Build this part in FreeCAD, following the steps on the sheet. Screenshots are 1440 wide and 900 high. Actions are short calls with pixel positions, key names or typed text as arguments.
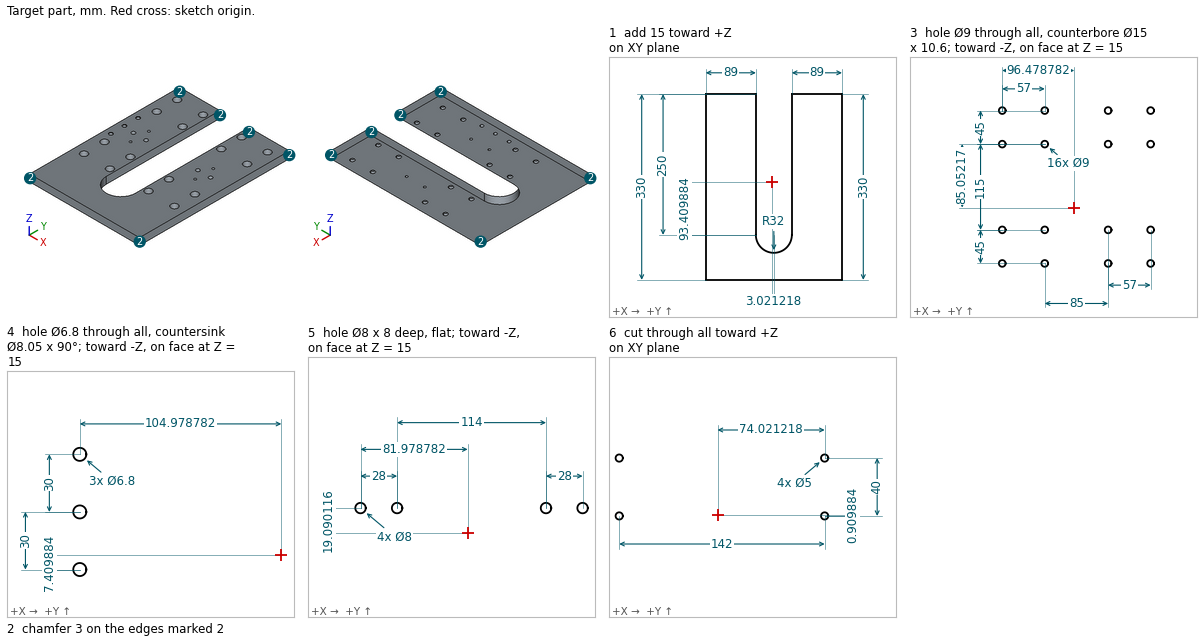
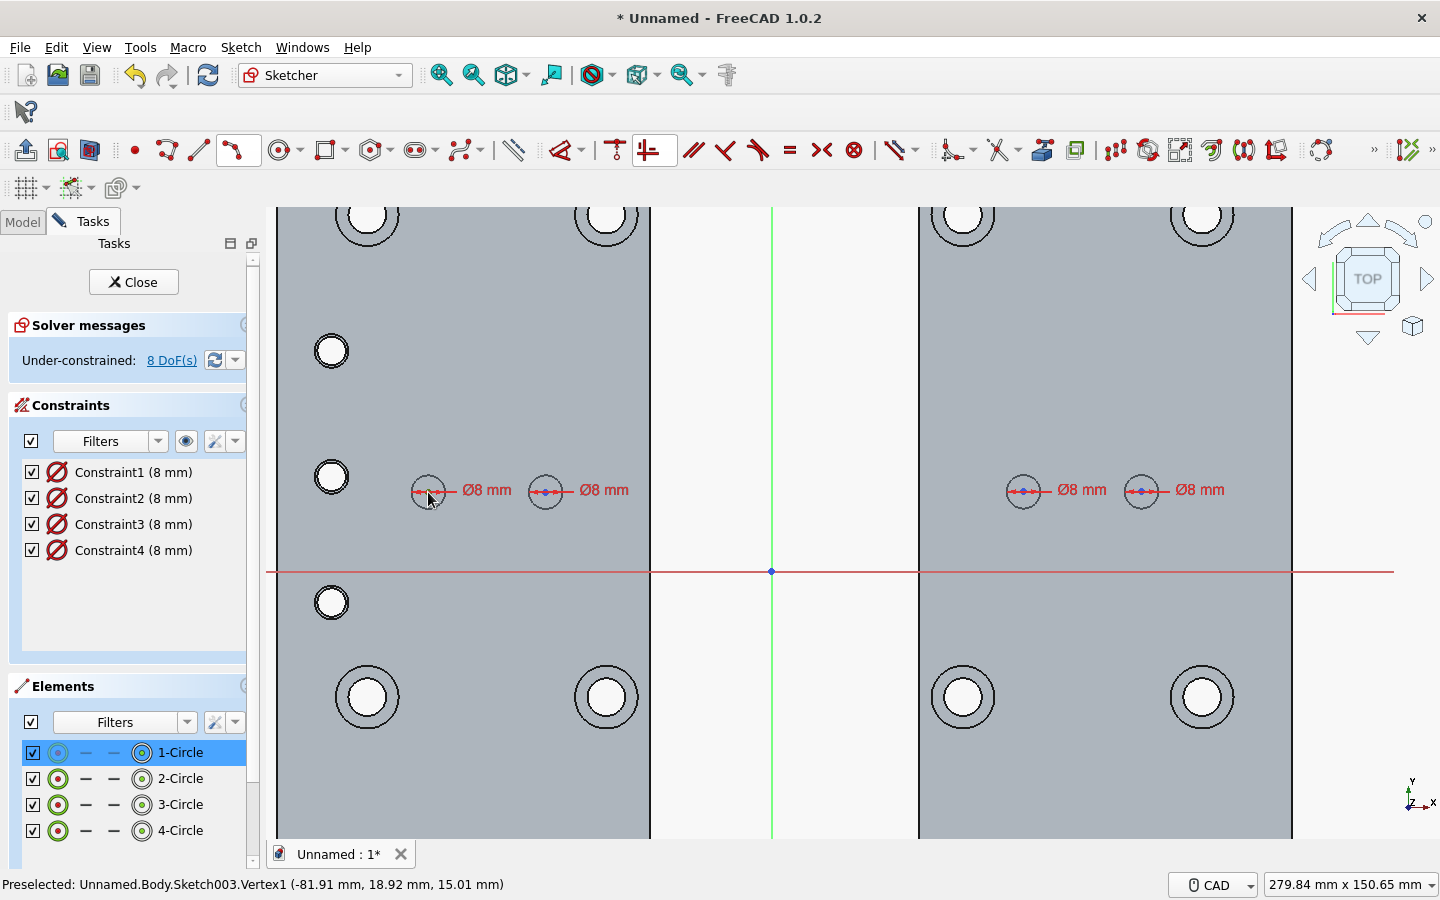
click(546, 492)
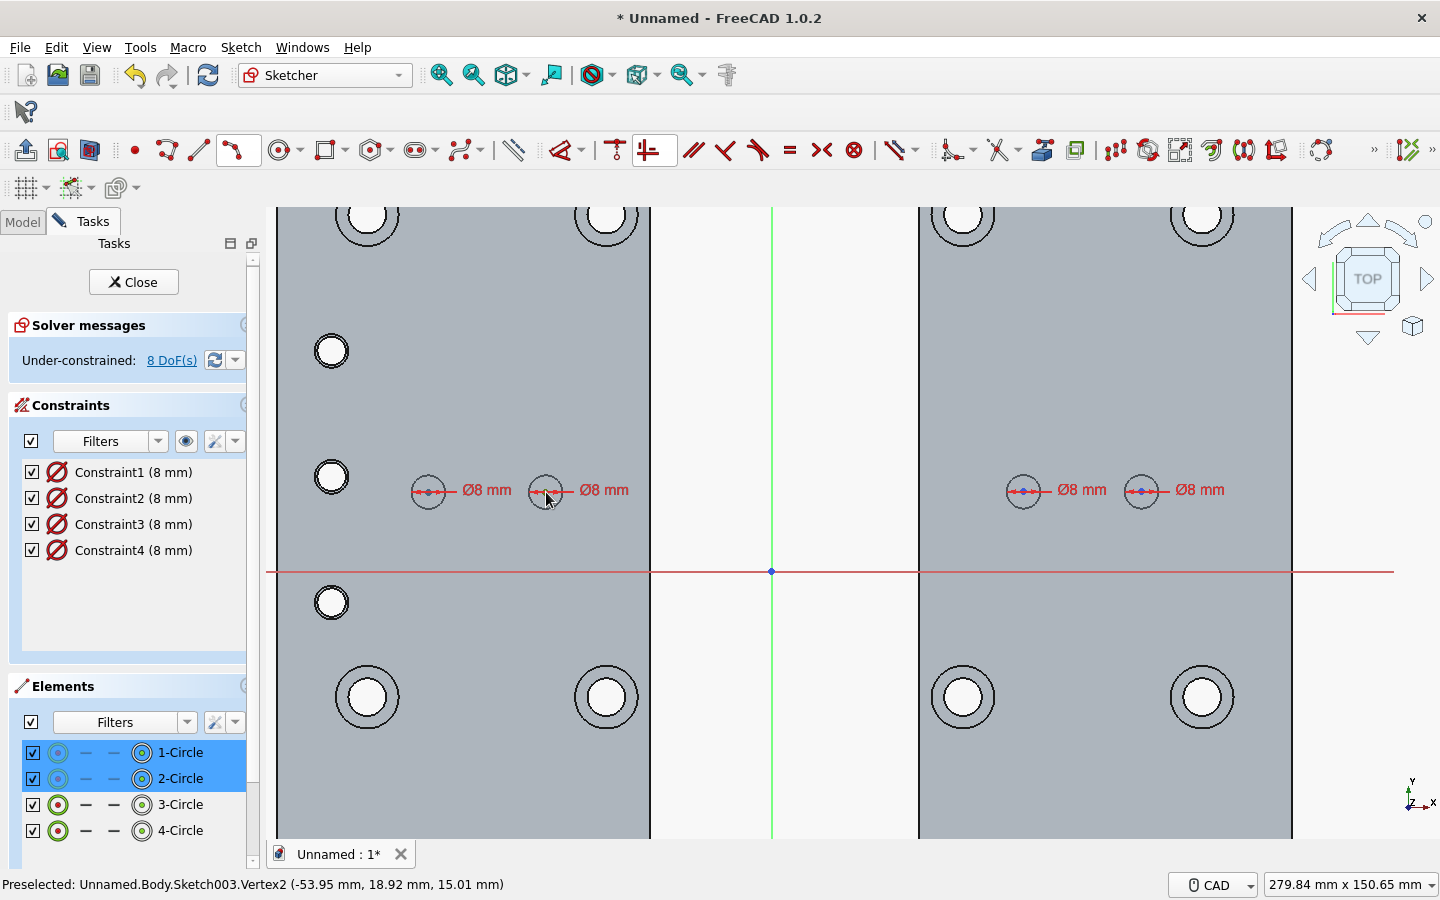
click(672, 150)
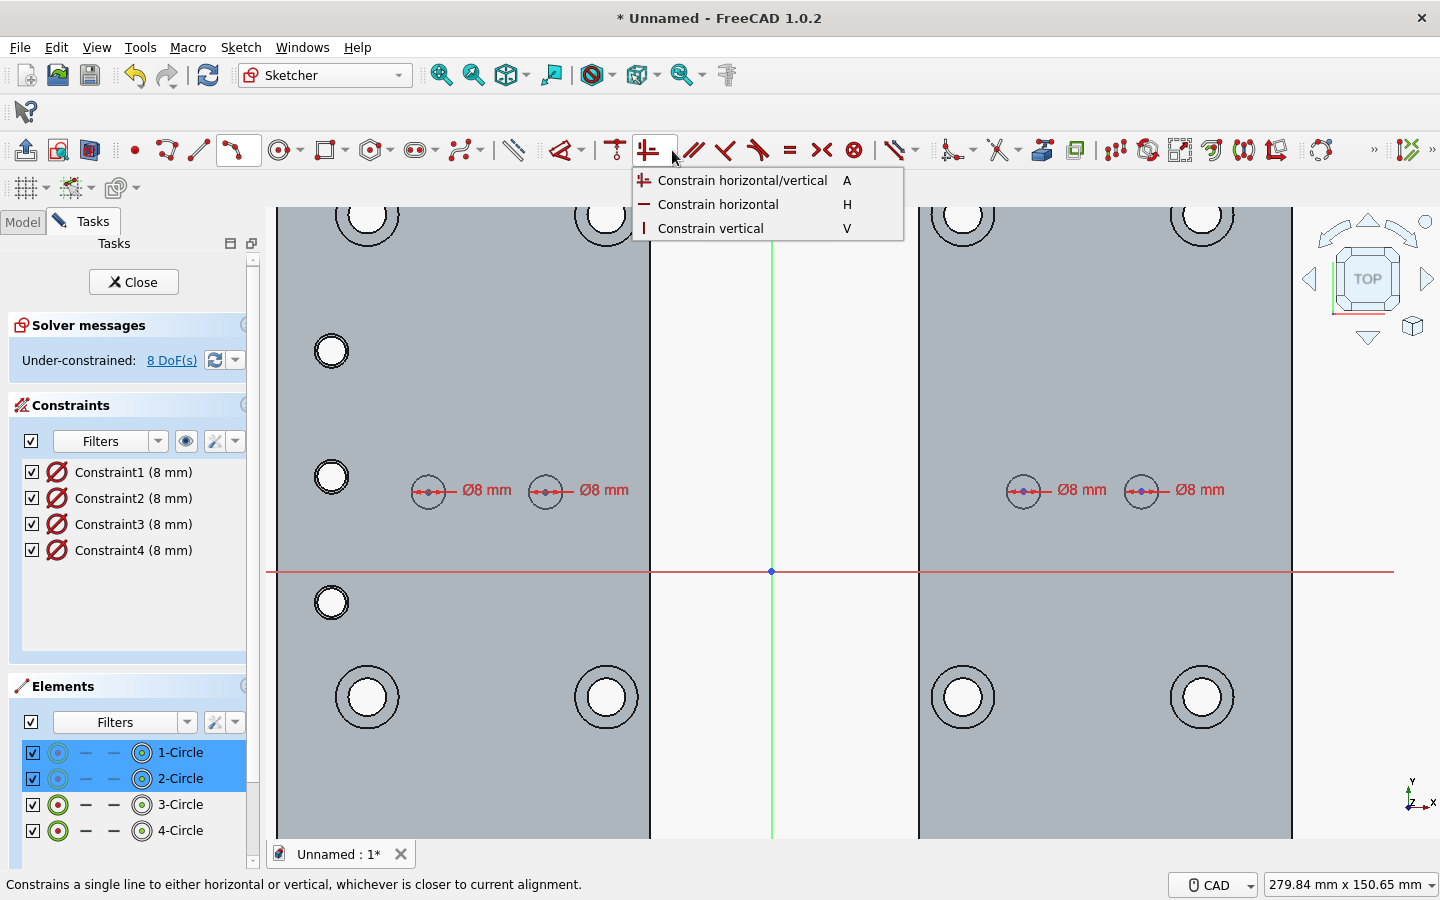
click(768, 204)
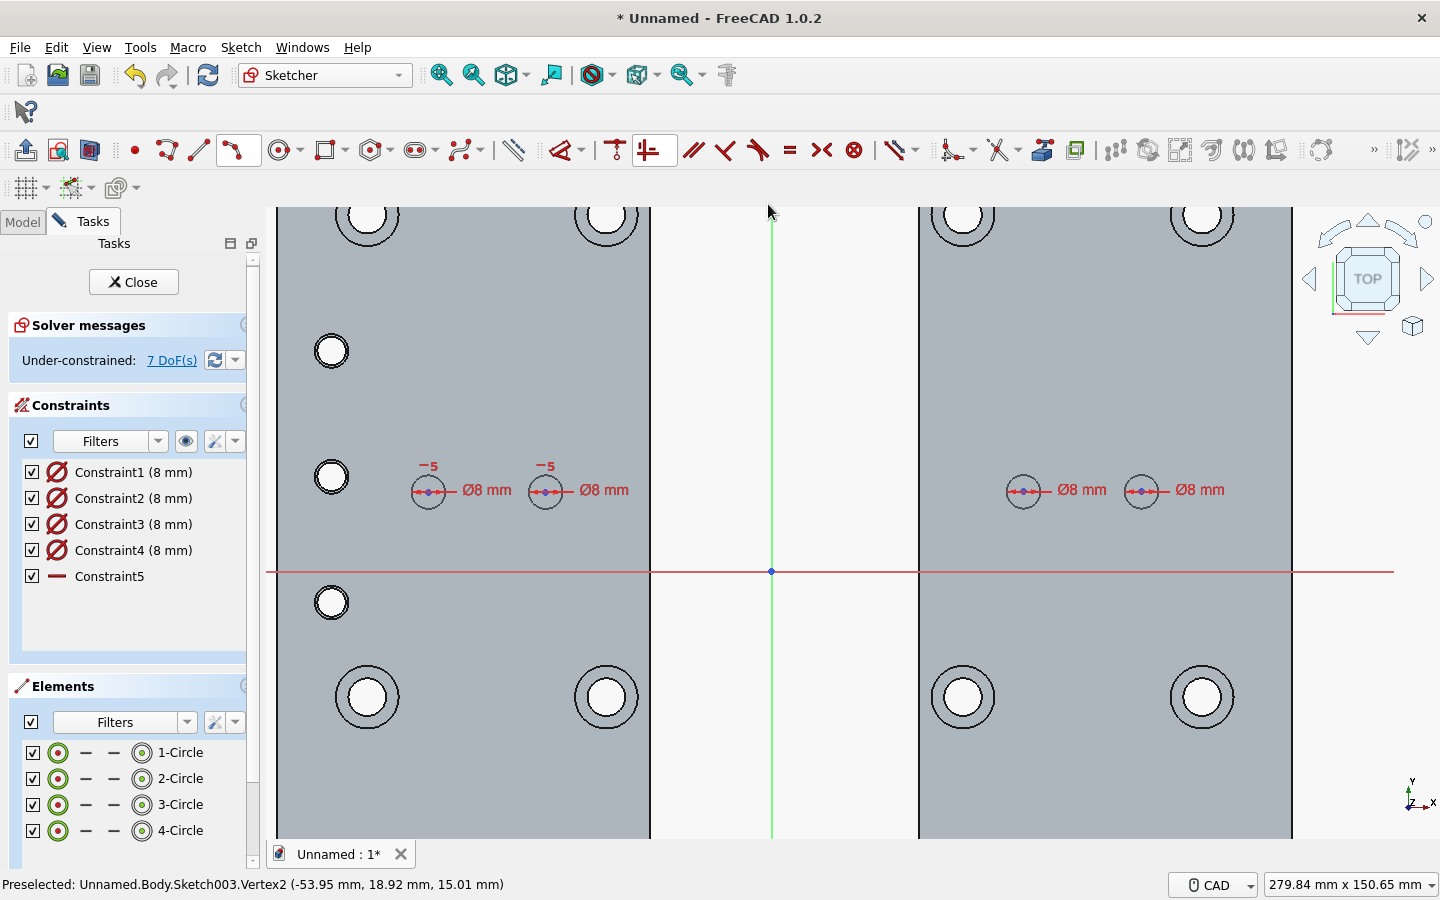
click(546, 492)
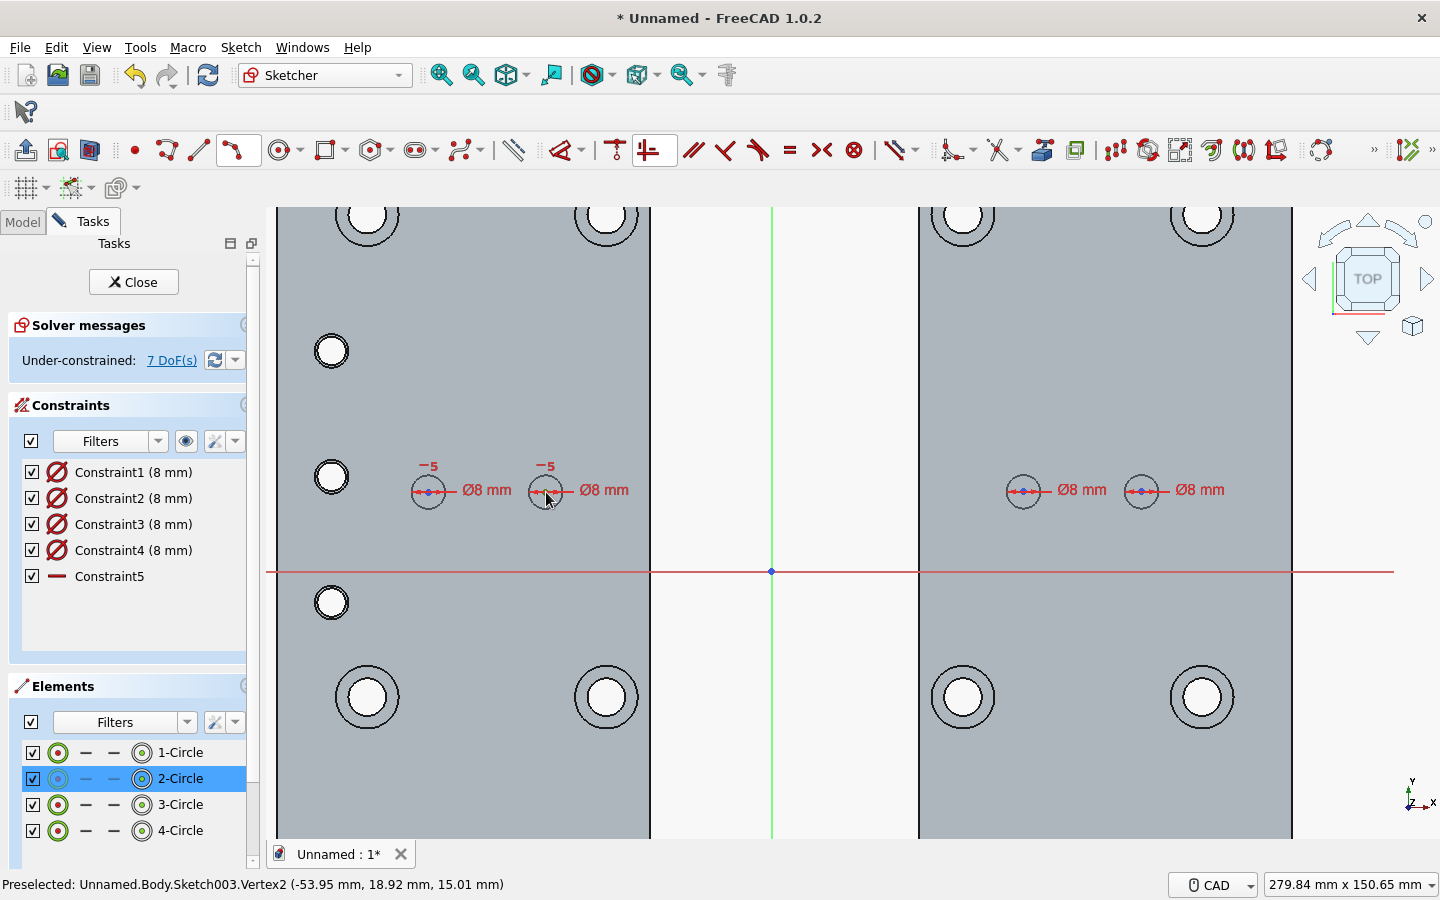
click(1024, 492)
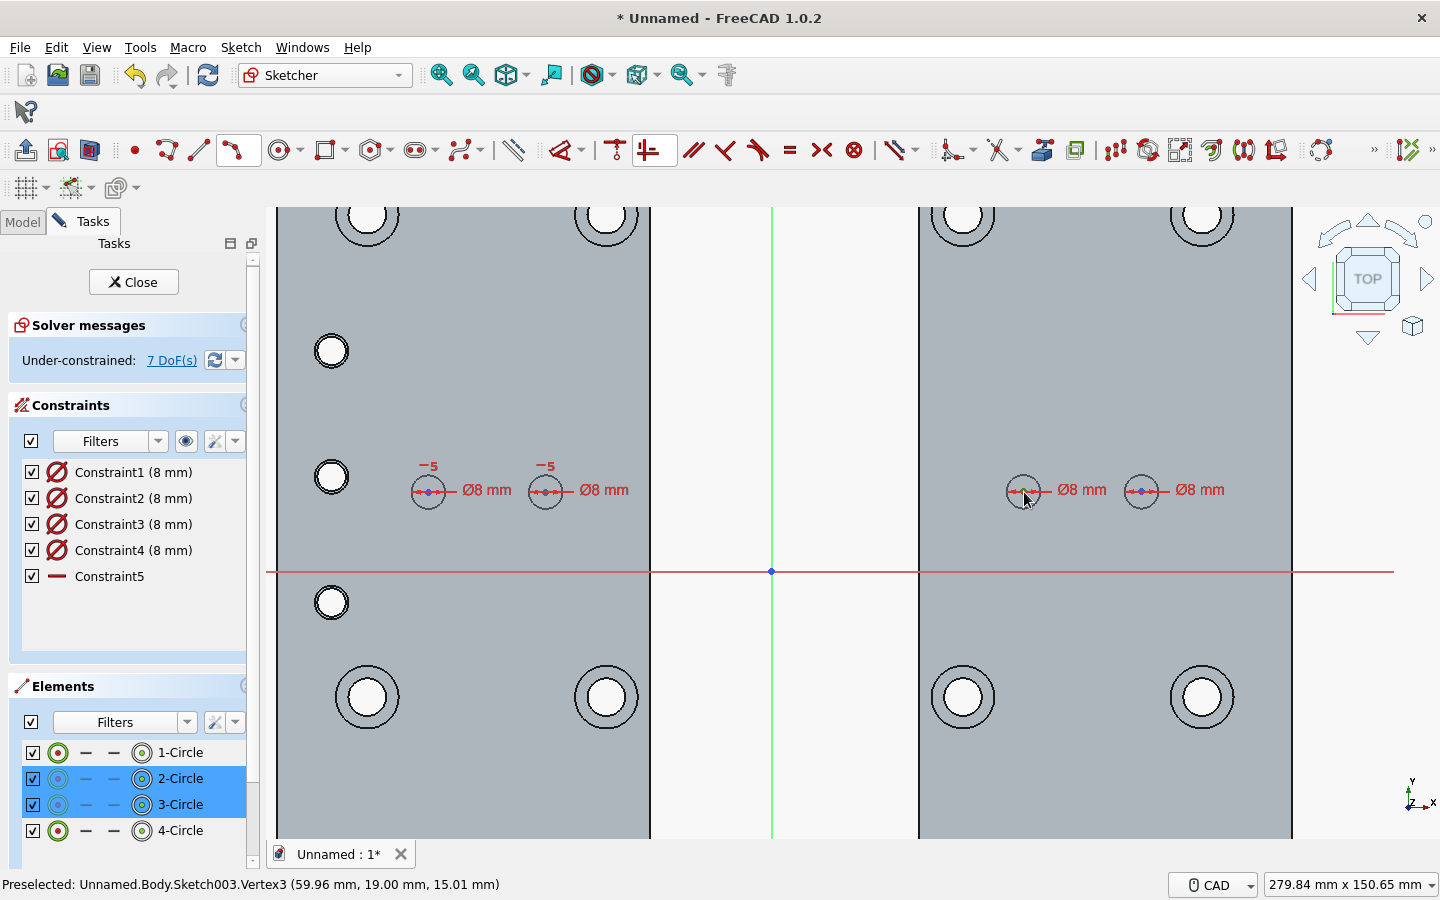
click(672, 150)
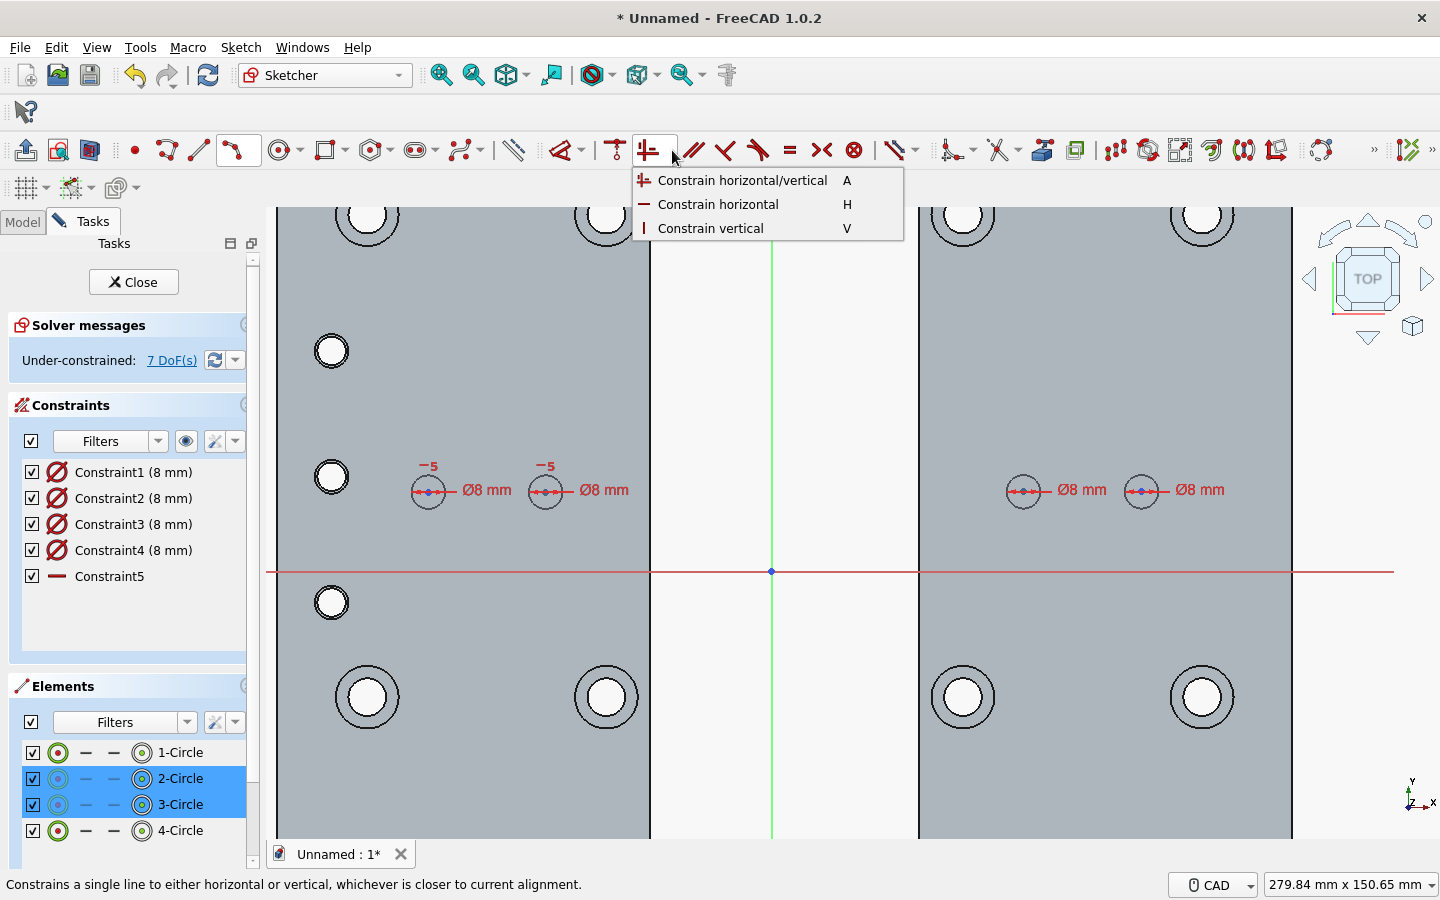
click(768, 204)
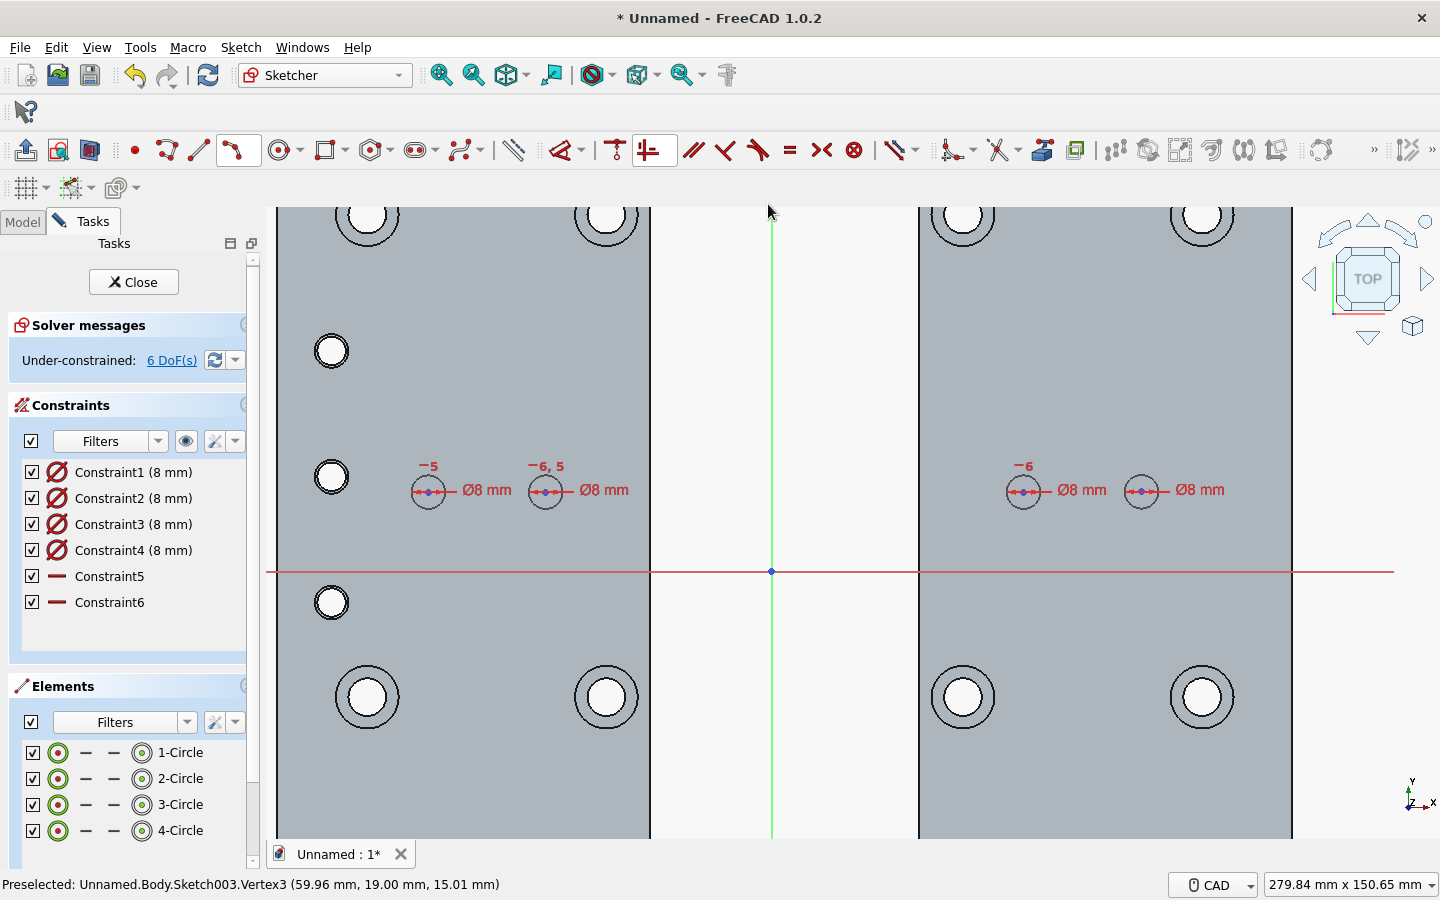
click(1024, 492)